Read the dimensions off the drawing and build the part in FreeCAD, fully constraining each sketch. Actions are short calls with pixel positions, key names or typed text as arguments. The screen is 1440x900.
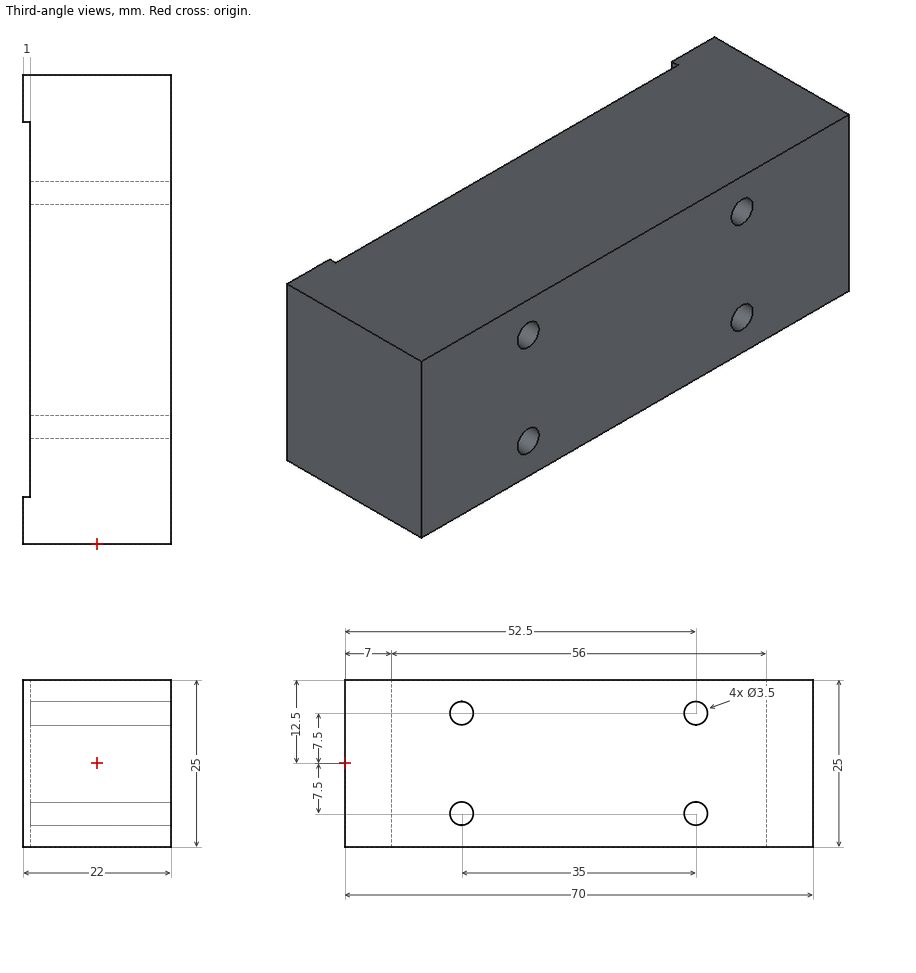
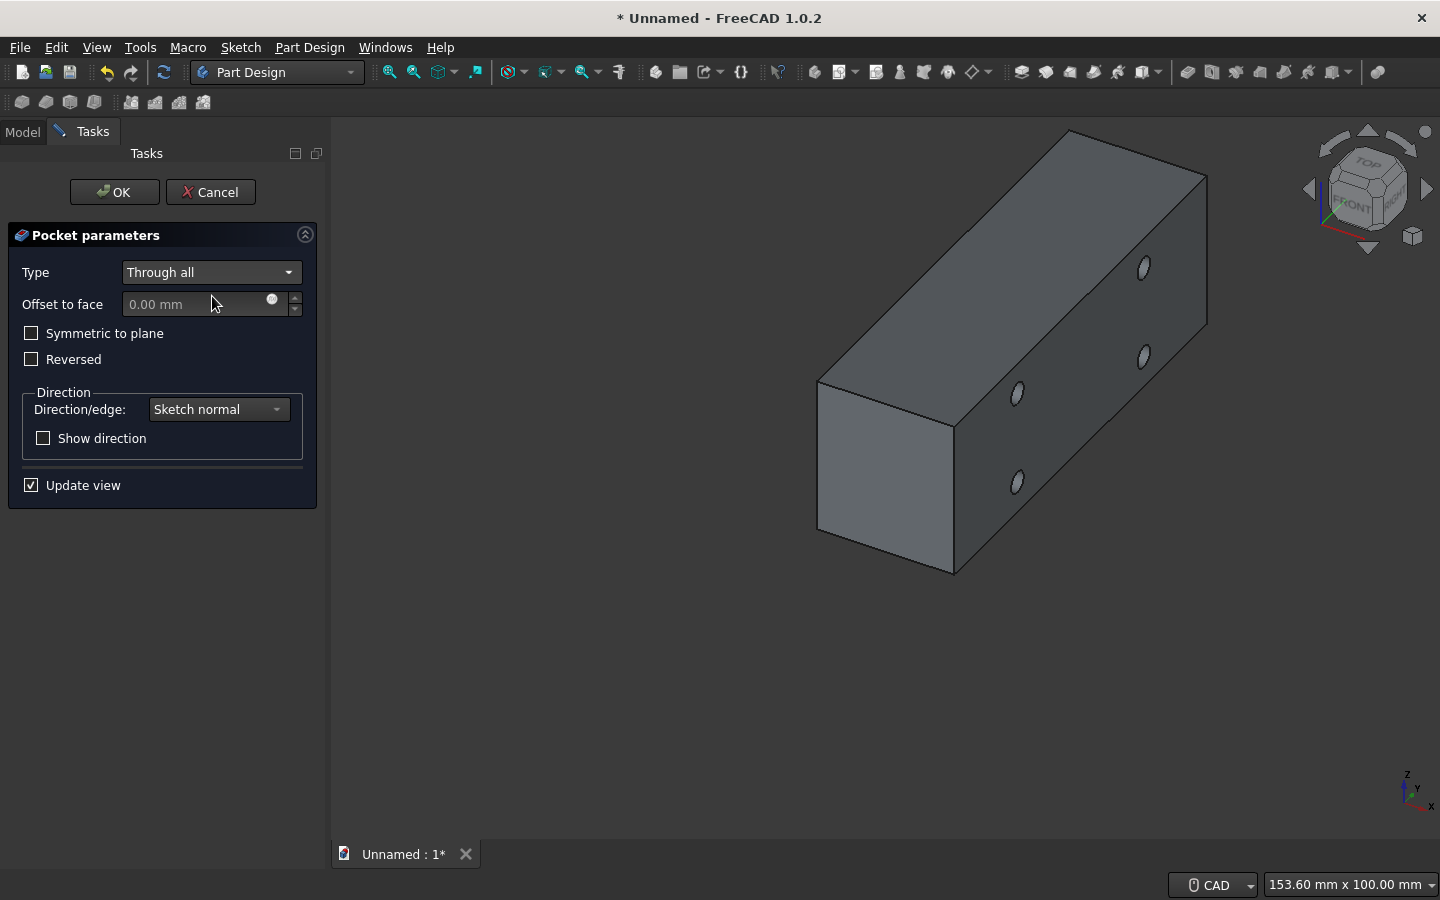
click(115, 192)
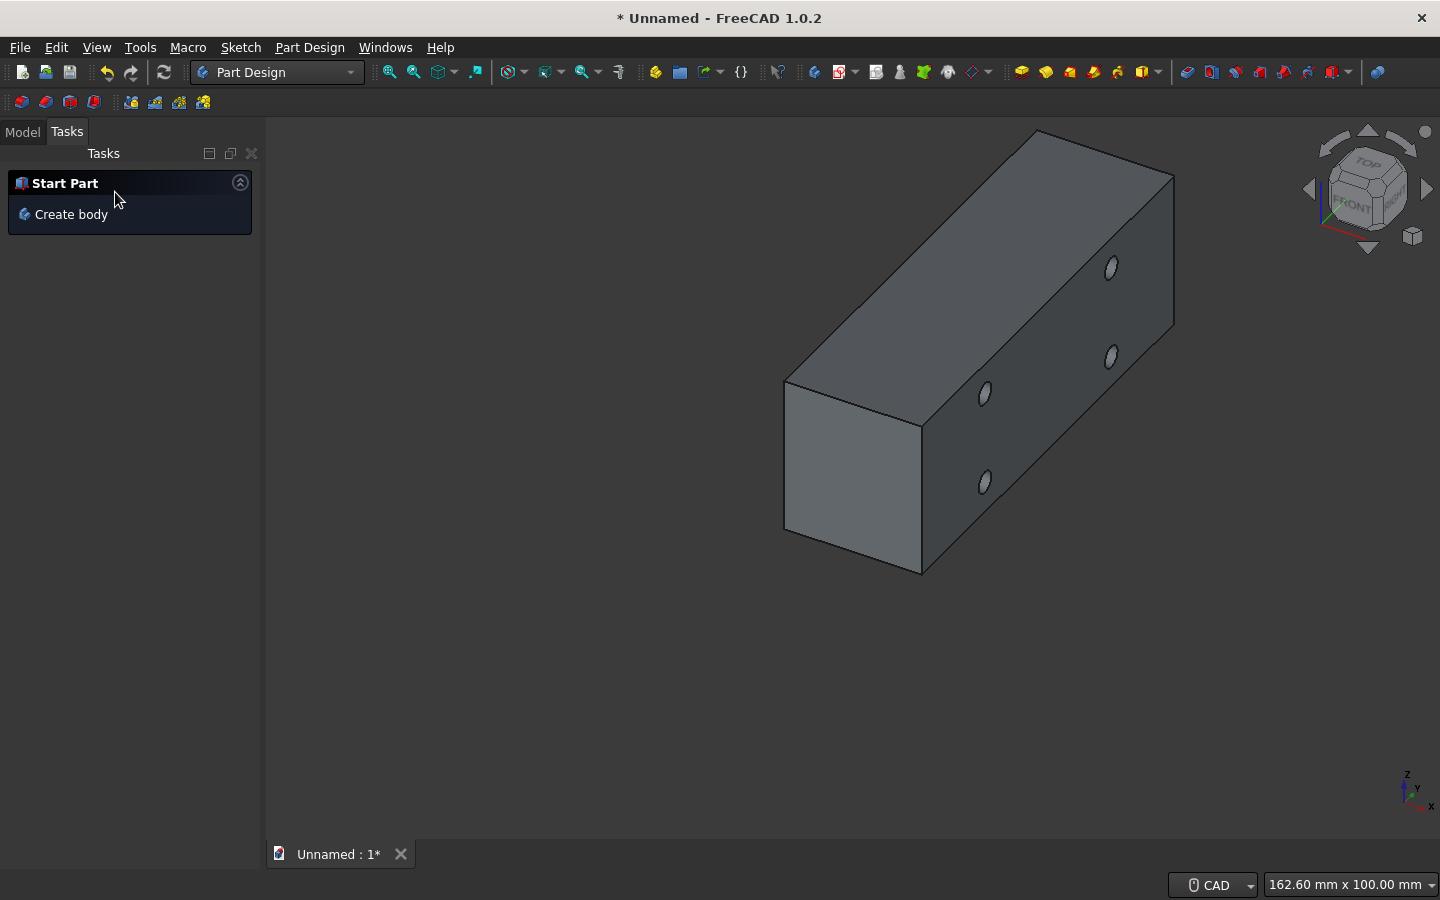
key(6)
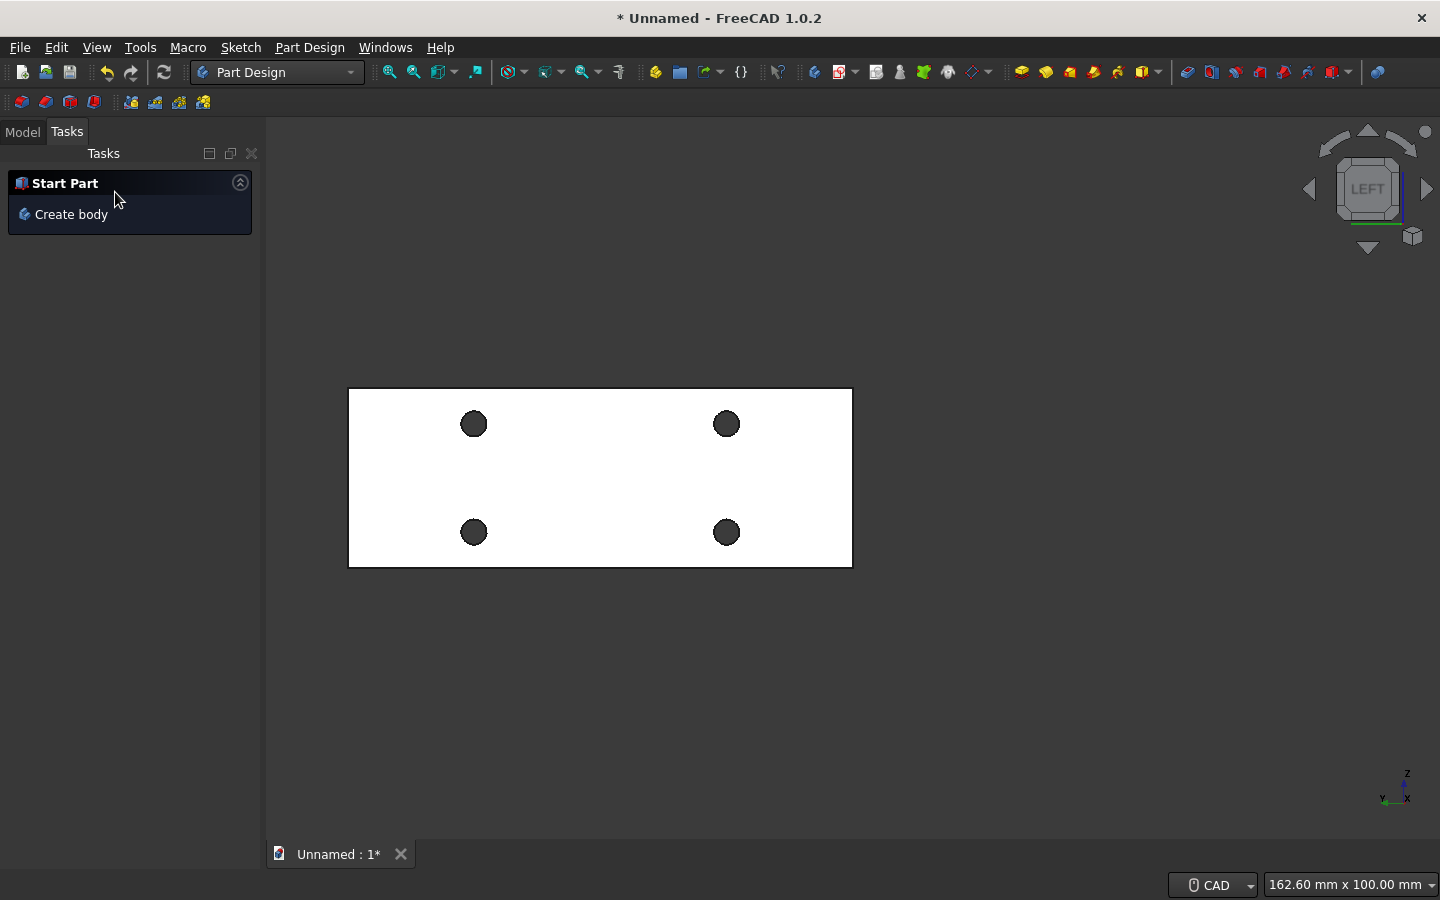
click(390, 72)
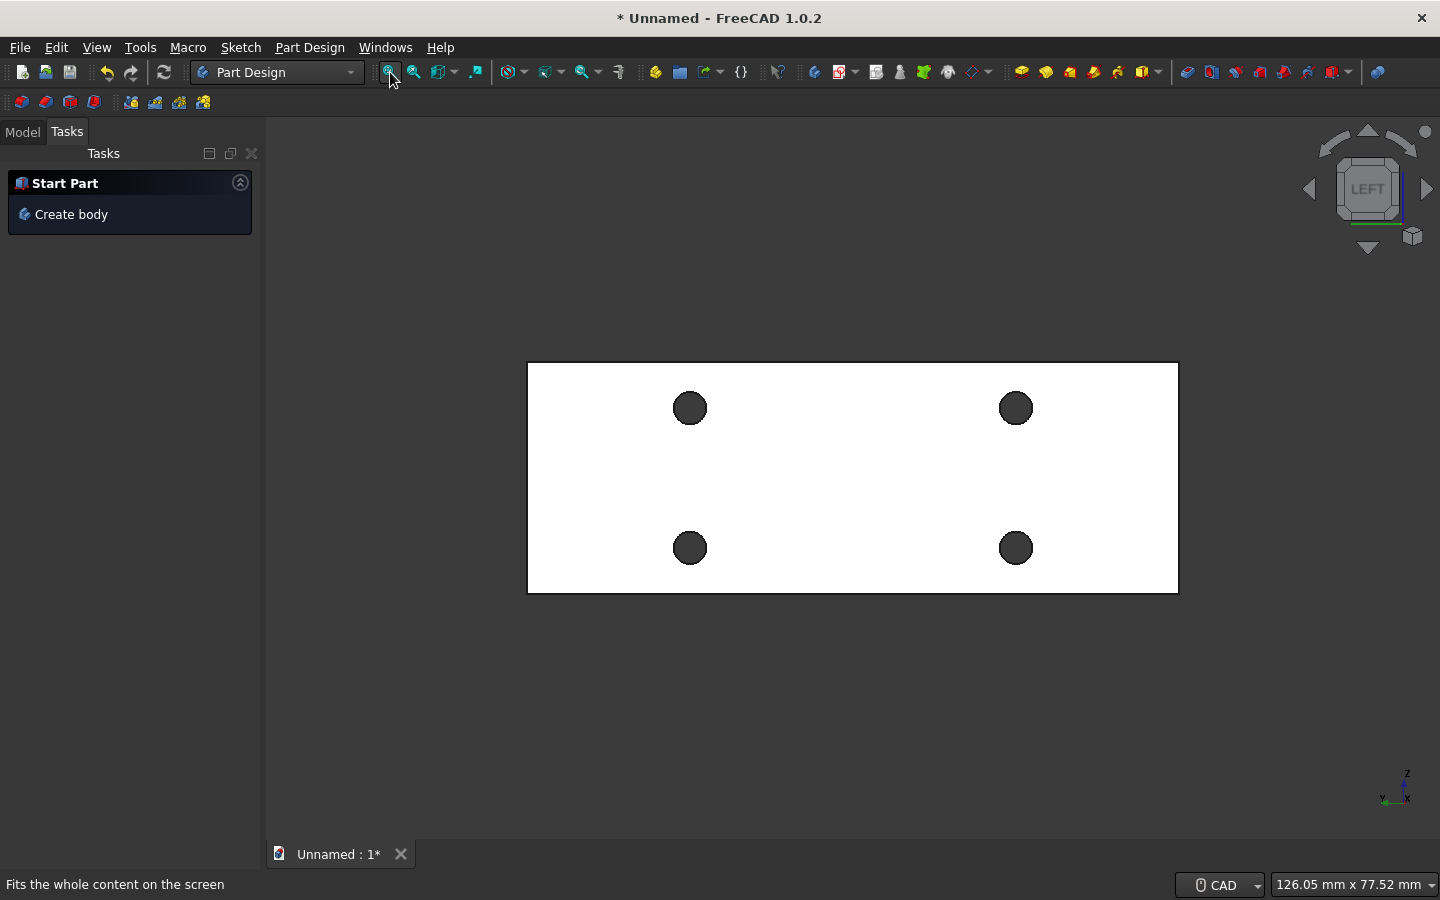
click(853, 477)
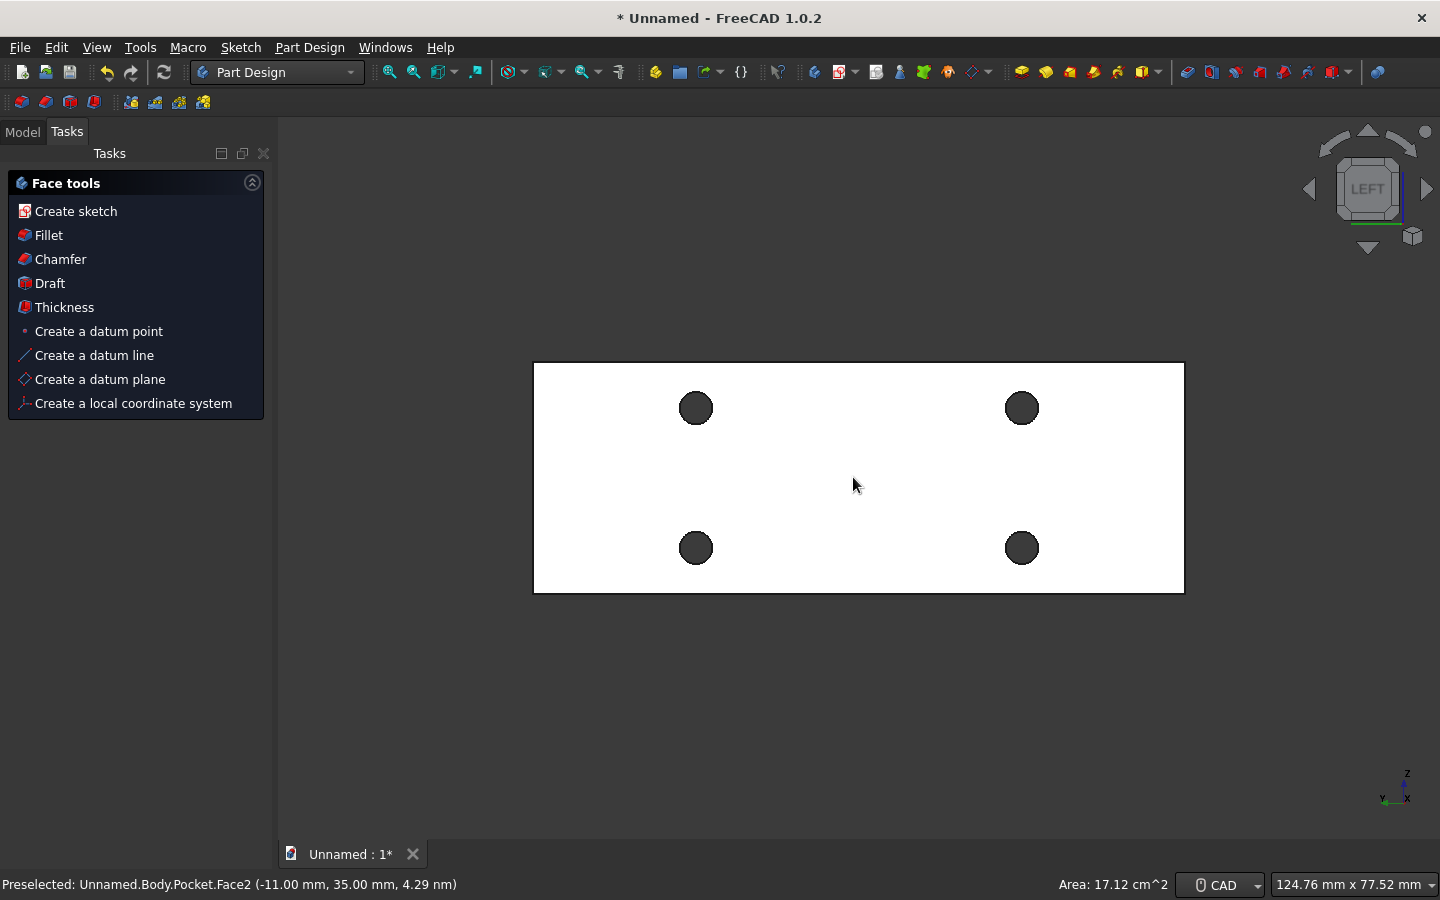
click(840, 72)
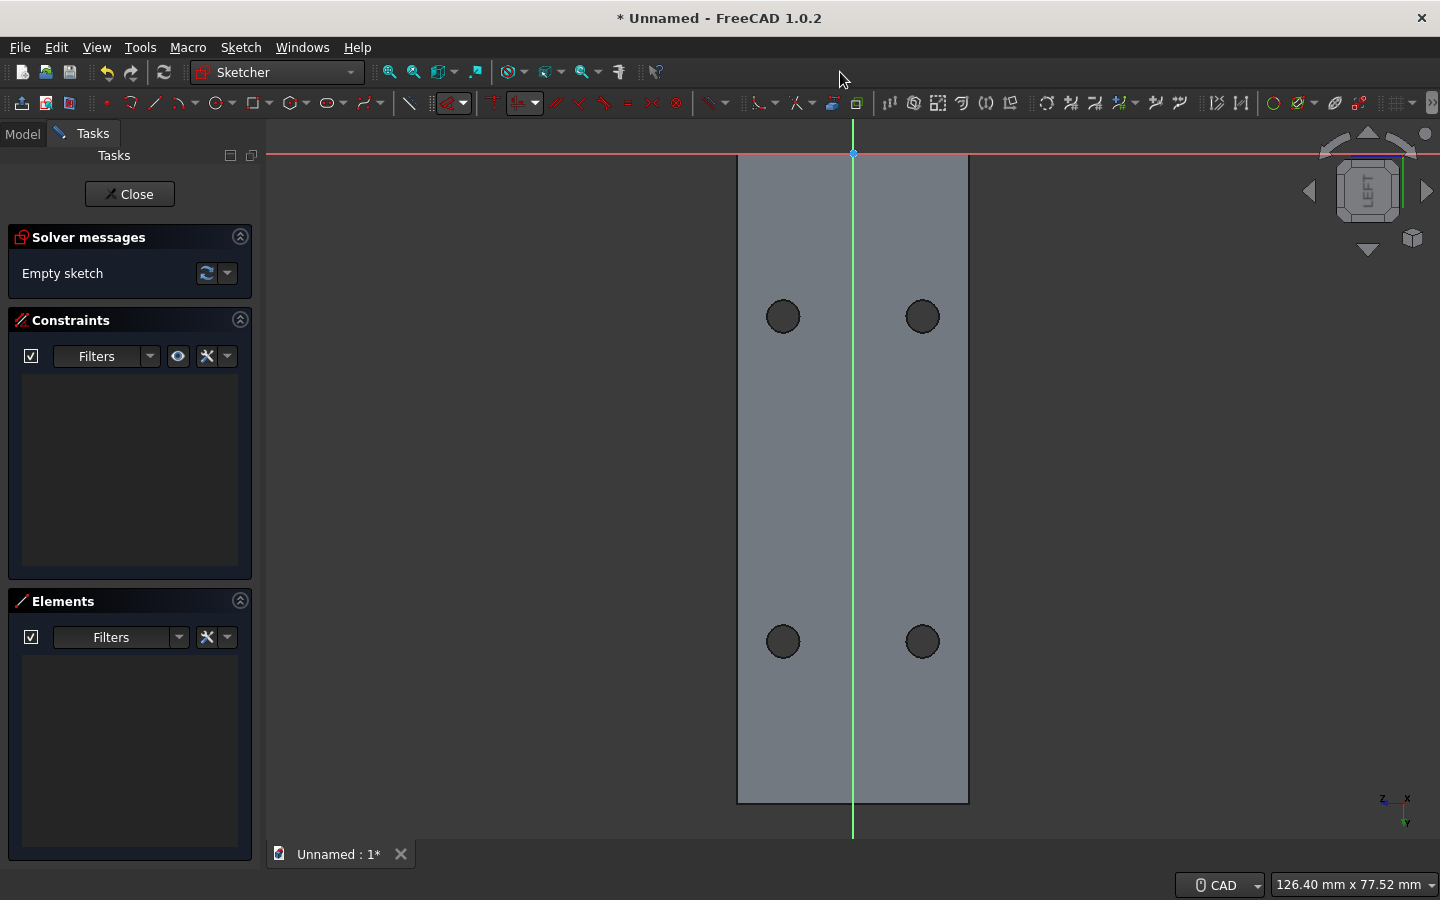
scroll(475, 626, down, 1)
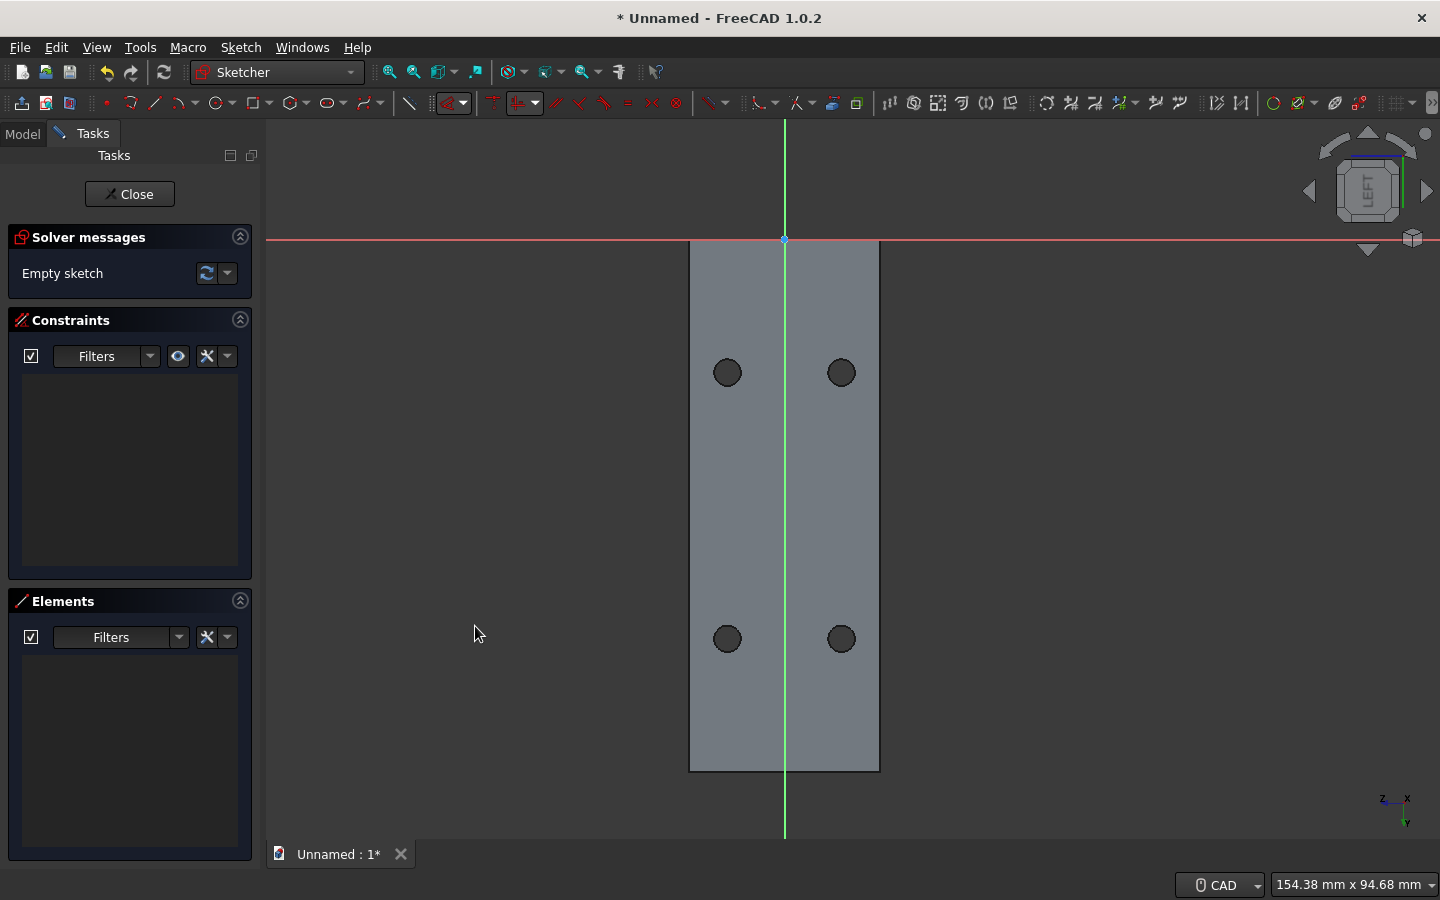
click(254, 104)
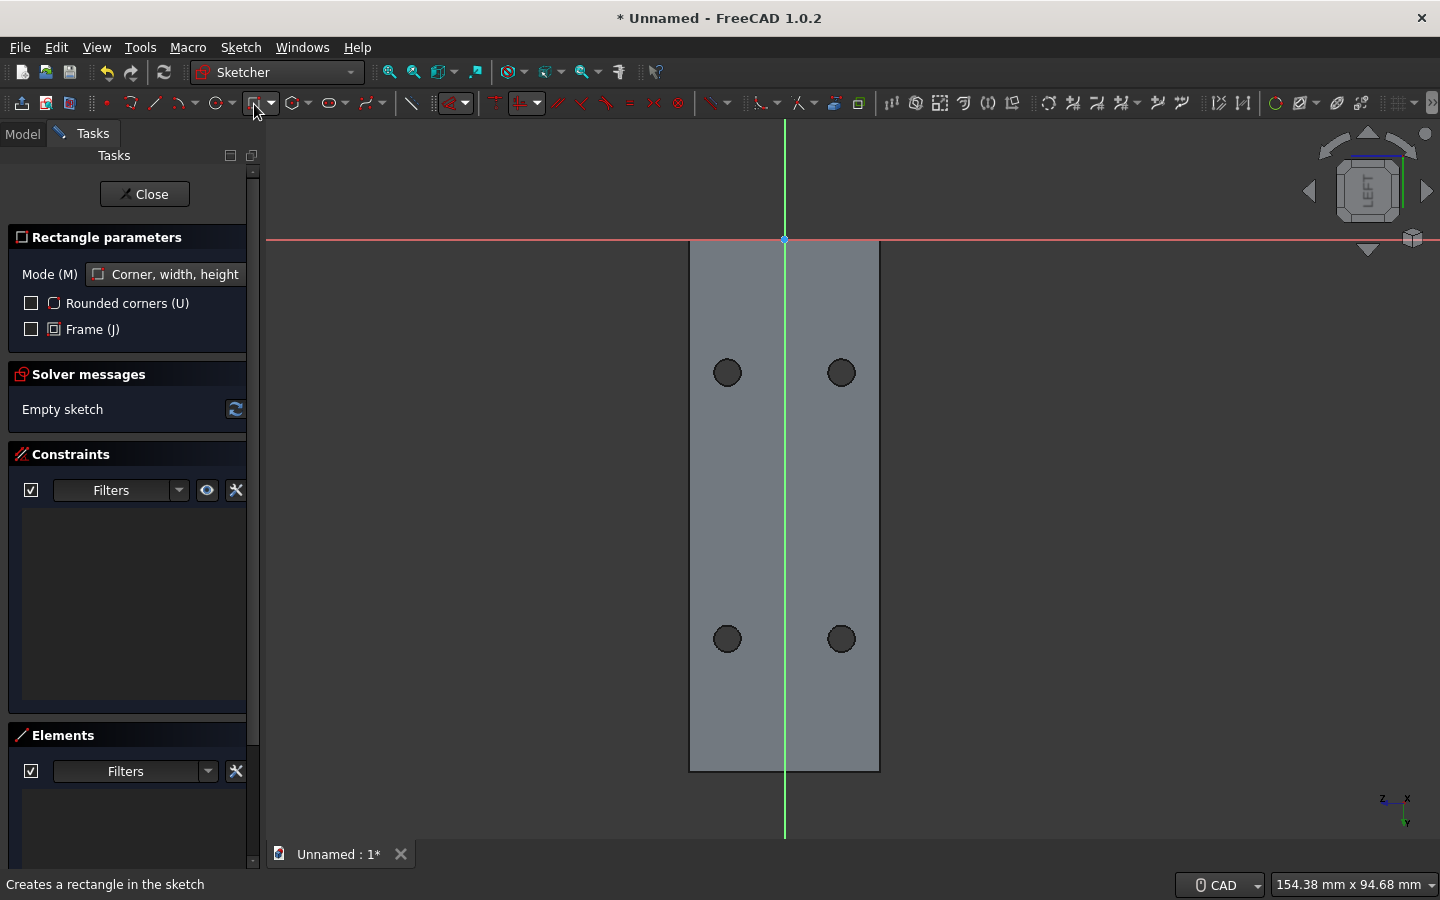
click(689, 293)
click(880, 719)
key(Escape)